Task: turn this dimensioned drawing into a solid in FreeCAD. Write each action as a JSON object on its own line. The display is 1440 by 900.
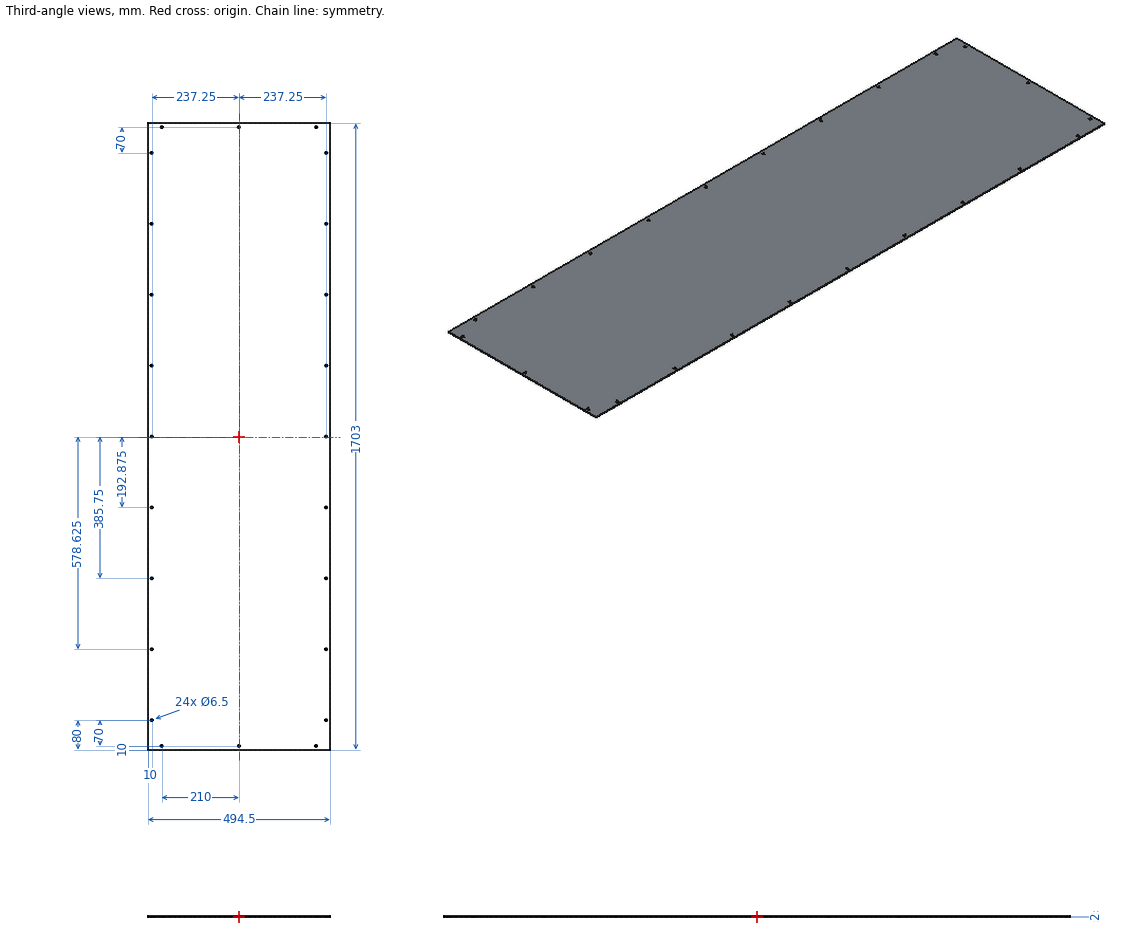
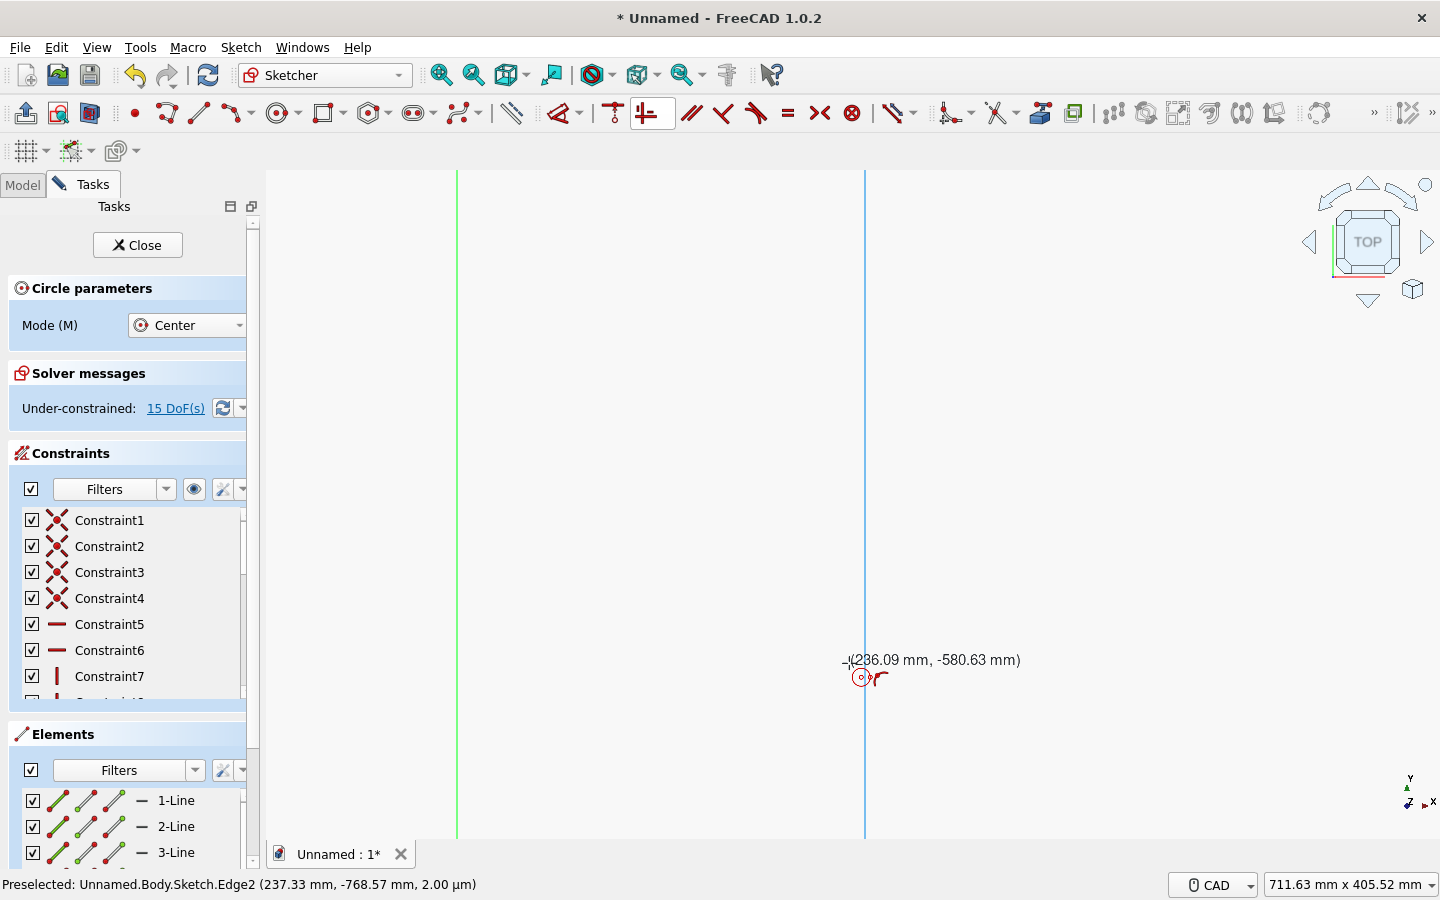
{"action": "left_click", "coordinate": [848, 662]}
{"action": "mouse_move", "coordinate": [845, 658]}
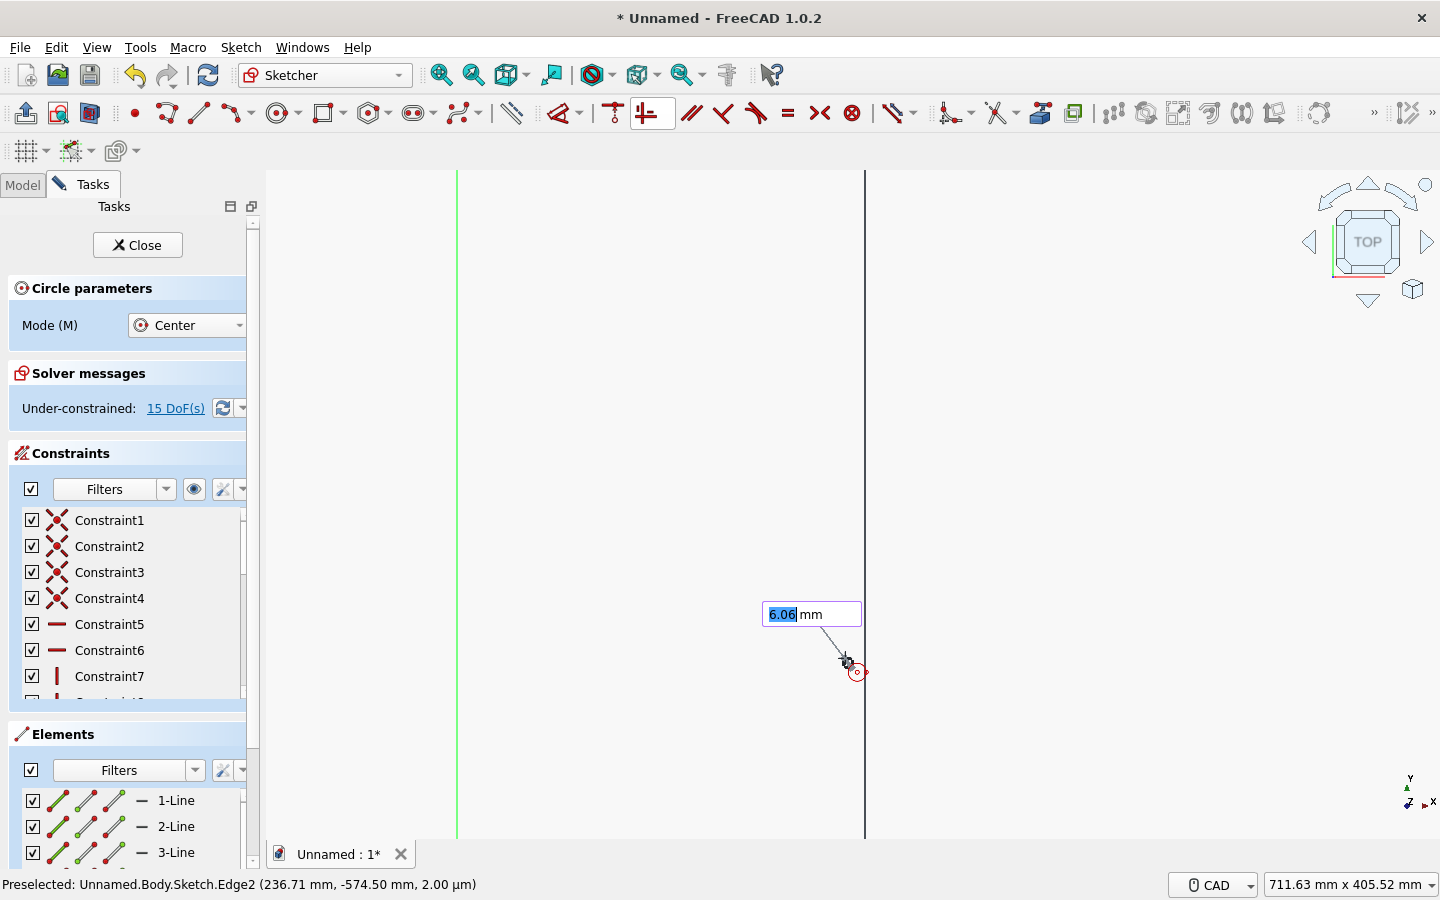
{"action": "type", "text": "6.5"}
{"action": "key", "text": "Return"}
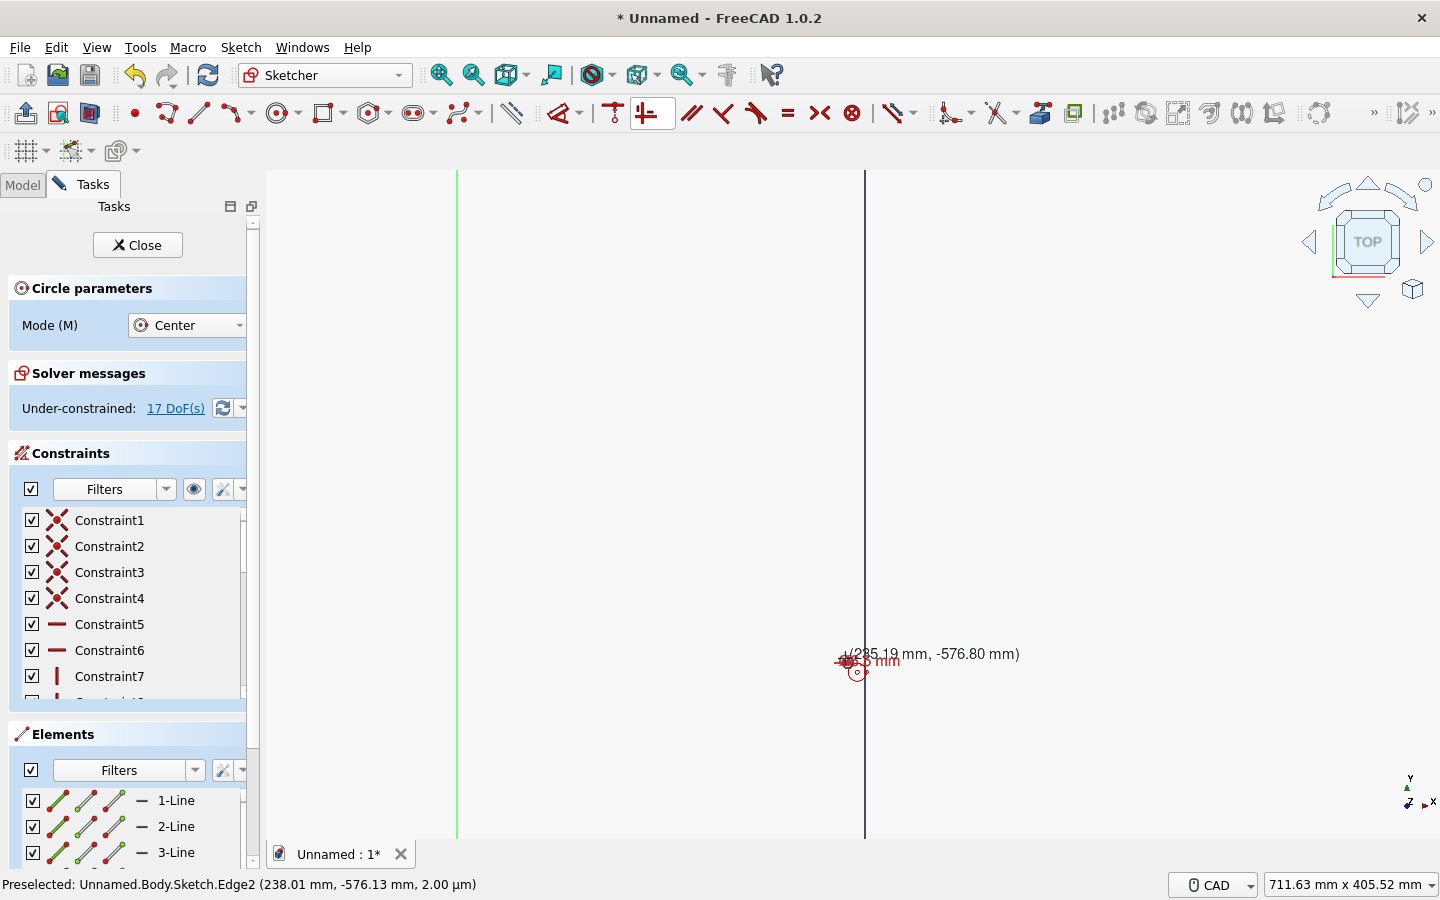
{"action": "scroll", "coordinate": [848, 344], "scroll_direction": "up", "scroll_amount": 8}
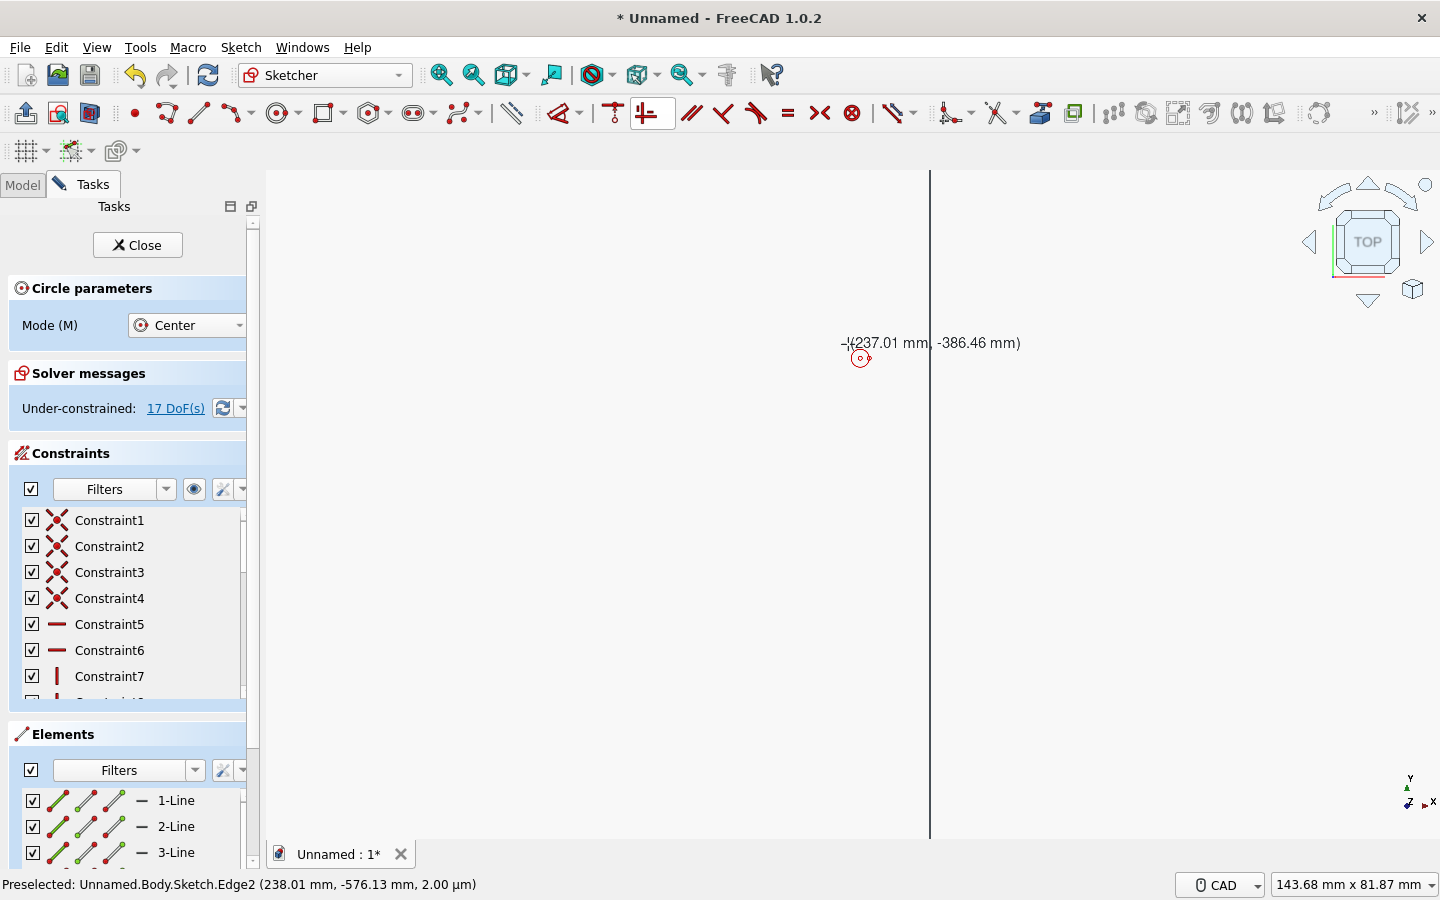
{"action": "scroll", "coordinate": [849, 619], "scroll_direction": "down", "scroll_amount": 17}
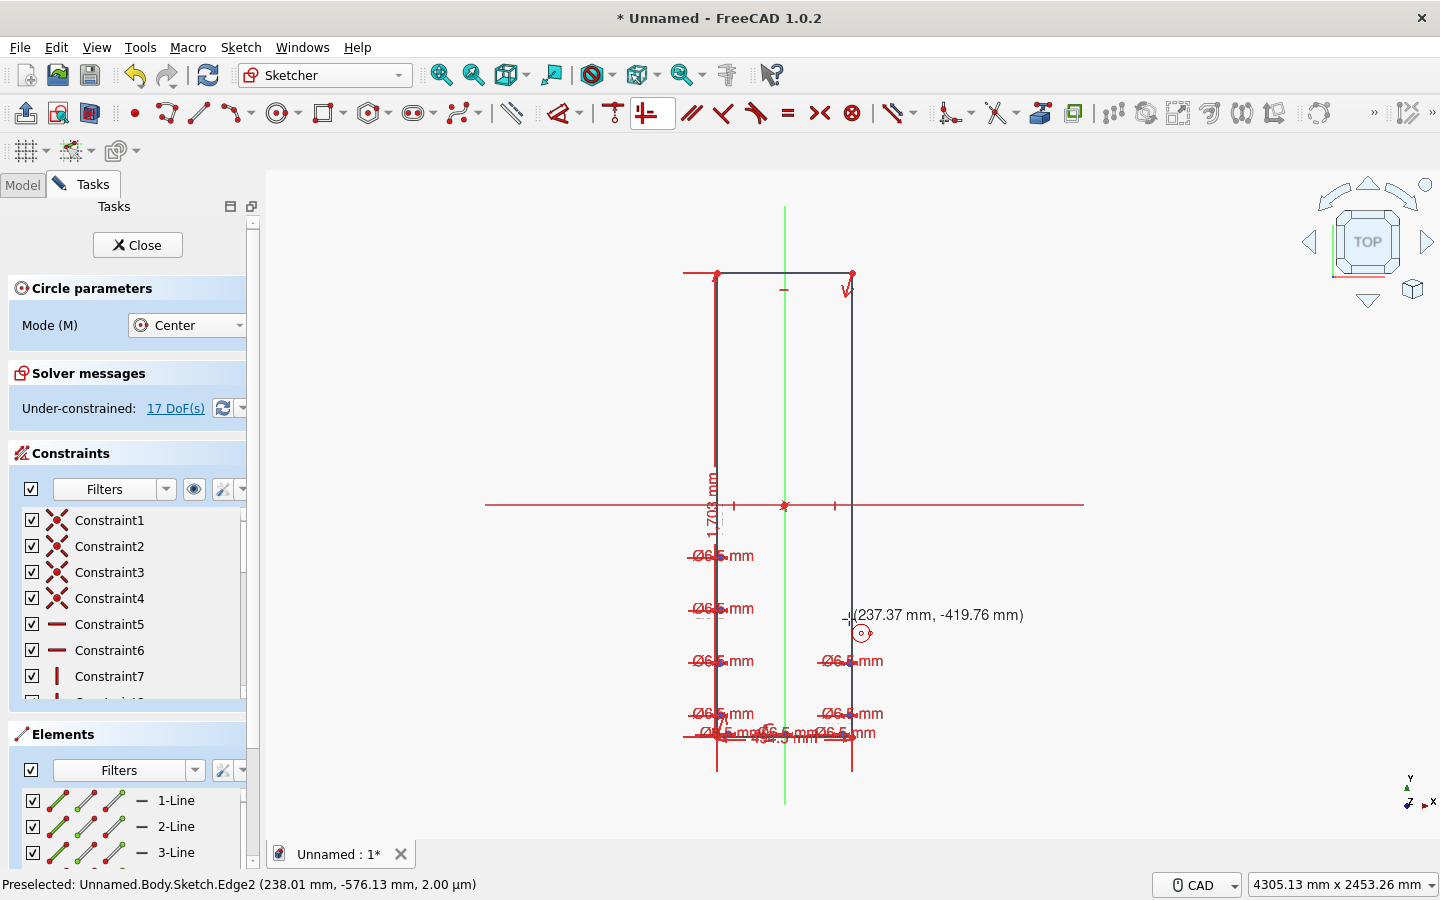
{"action": "scroll", "coordinate": [849, 610], "scroll_direction": "up", "scroll_amount": 9}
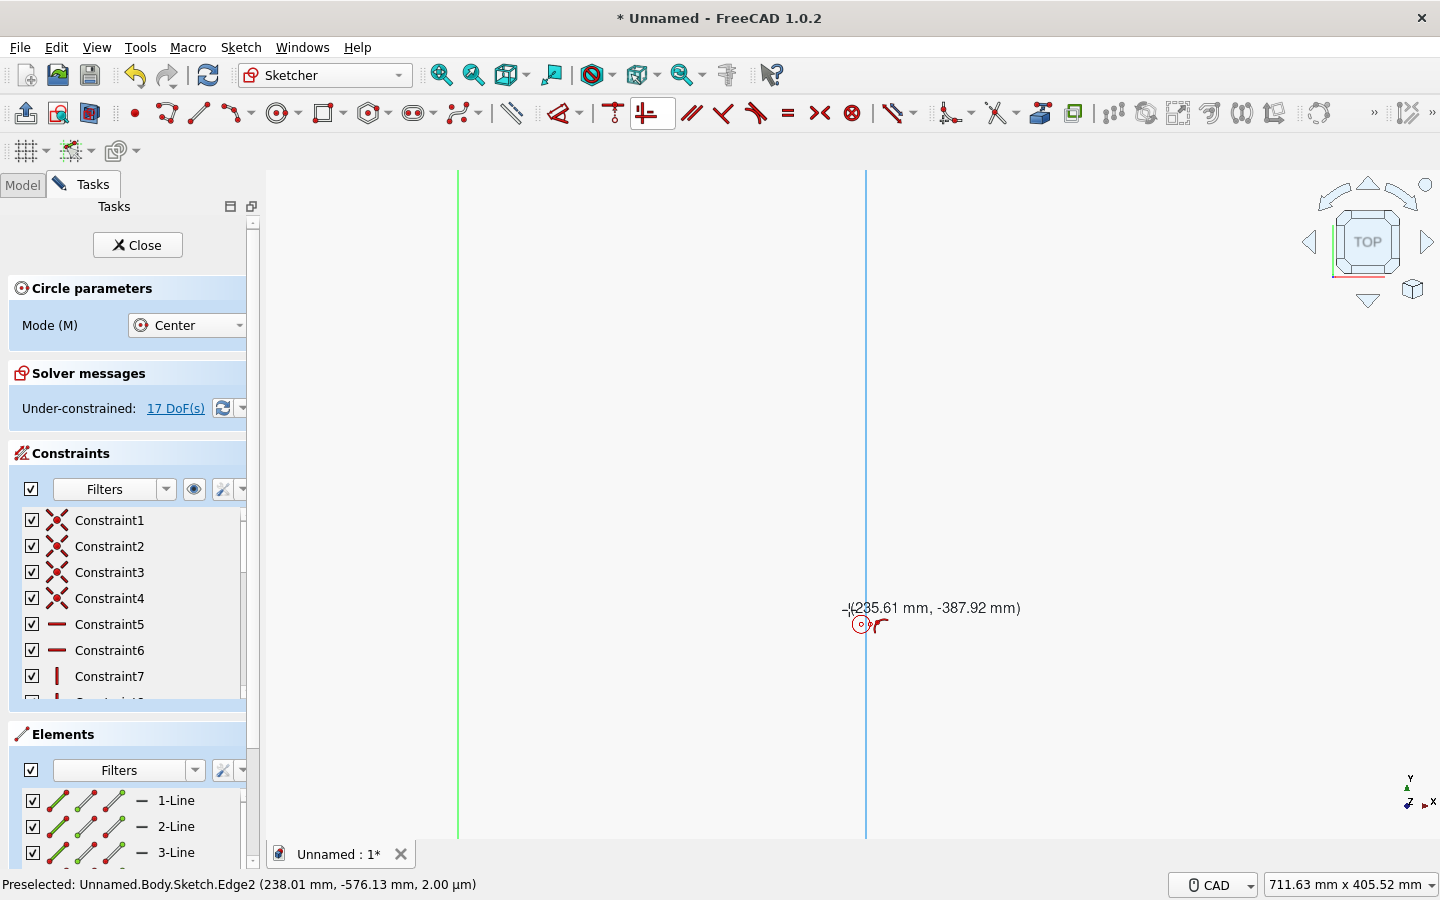
{"action": "left_click", "coordinate": [849, 609]}
{"action": "mouse_move", "coordinate": [845, 605]}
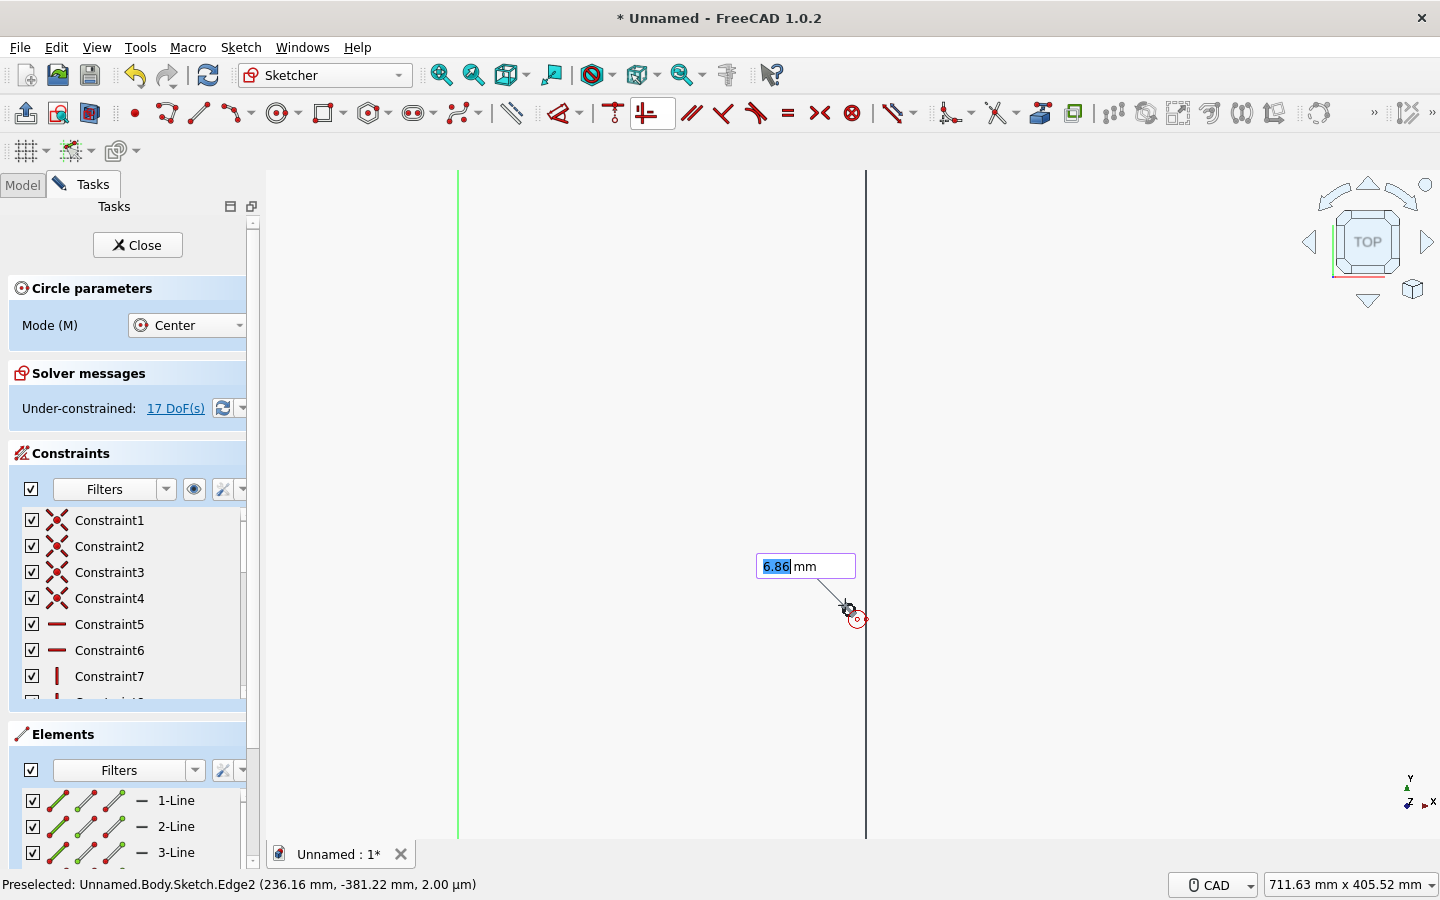
{"action": "type", "text": "6.5"}
{"action": "key", "text": "Return"}